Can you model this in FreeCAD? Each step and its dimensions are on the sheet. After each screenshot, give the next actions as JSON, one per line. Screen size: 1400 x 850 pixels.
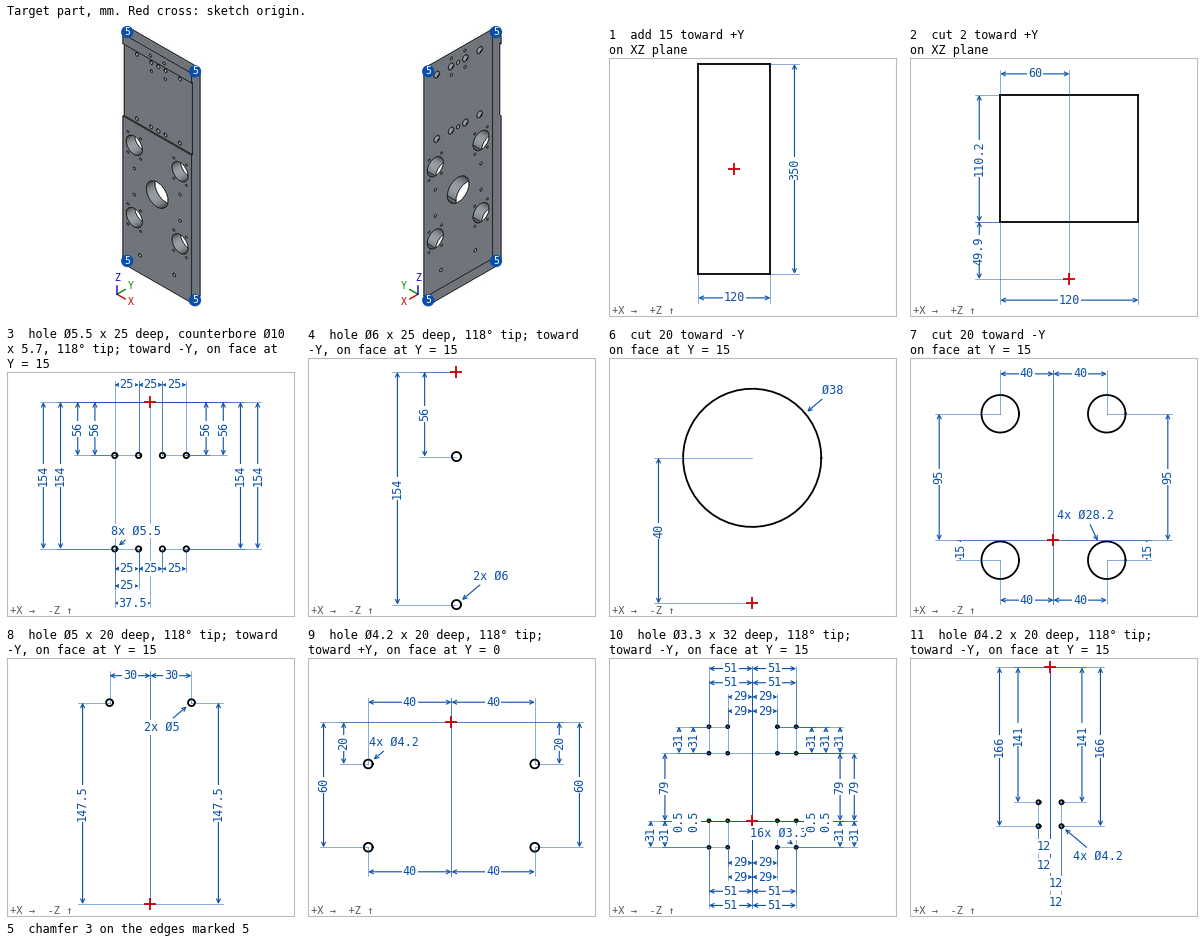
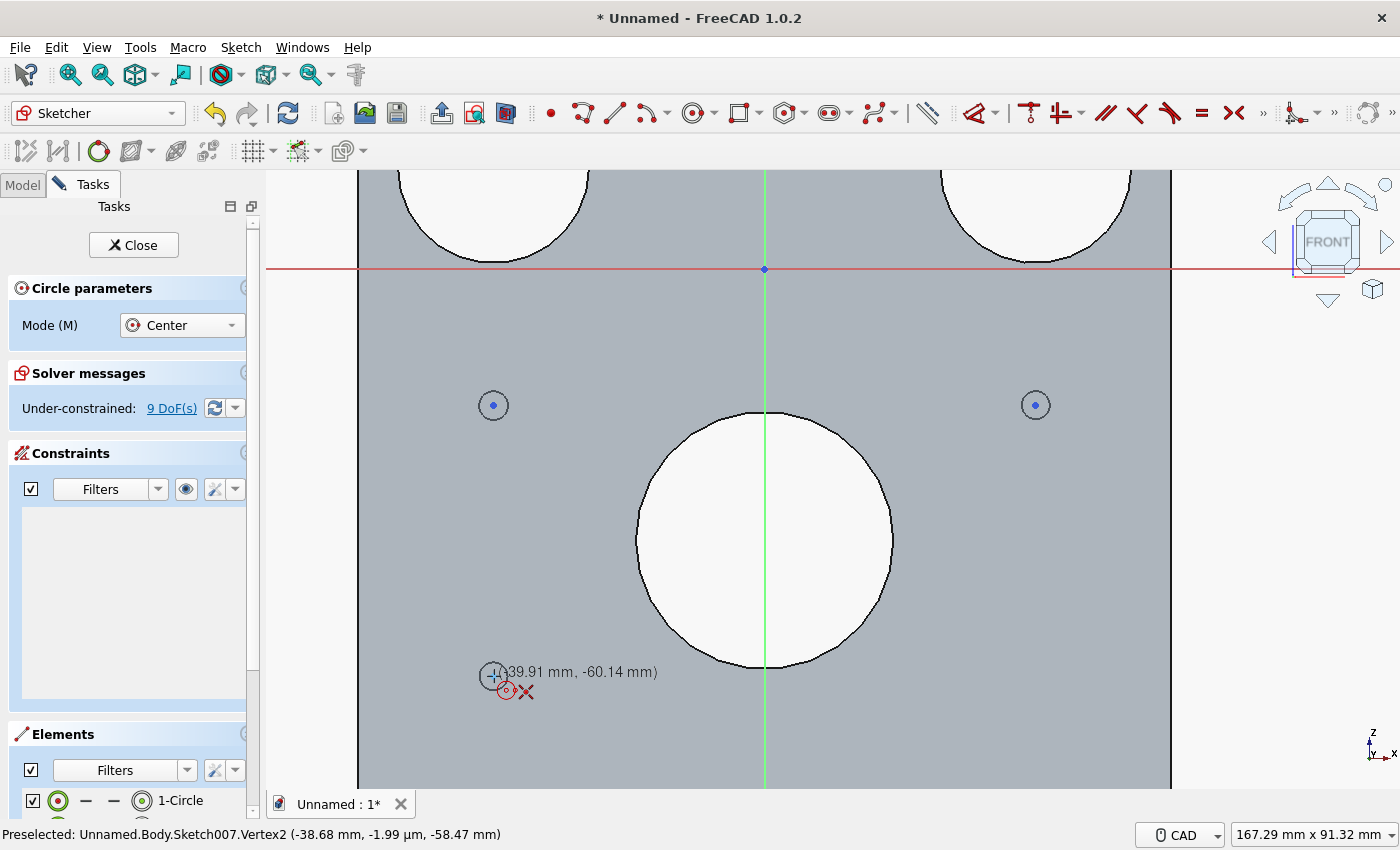
{"action": "scroll", "coordinate": [1036, 676], "scroll_direction": "up", "scroll_amount": 3}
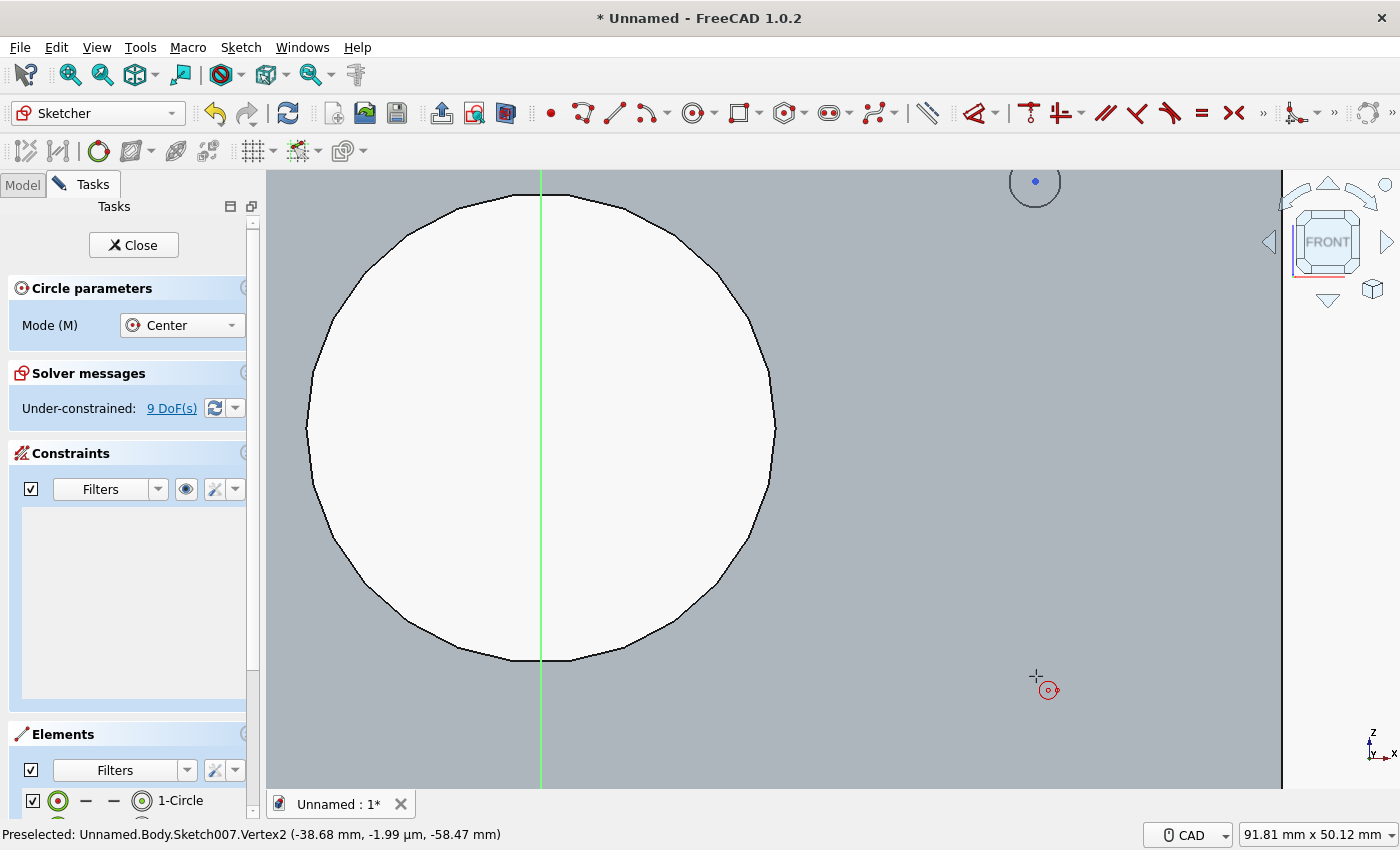
{"action": "left_click", "coordinate": [1035, 675]}
{"action": "left_click", "coordinate": [1053, 657]}
{"action": "key", "text": "Escape"}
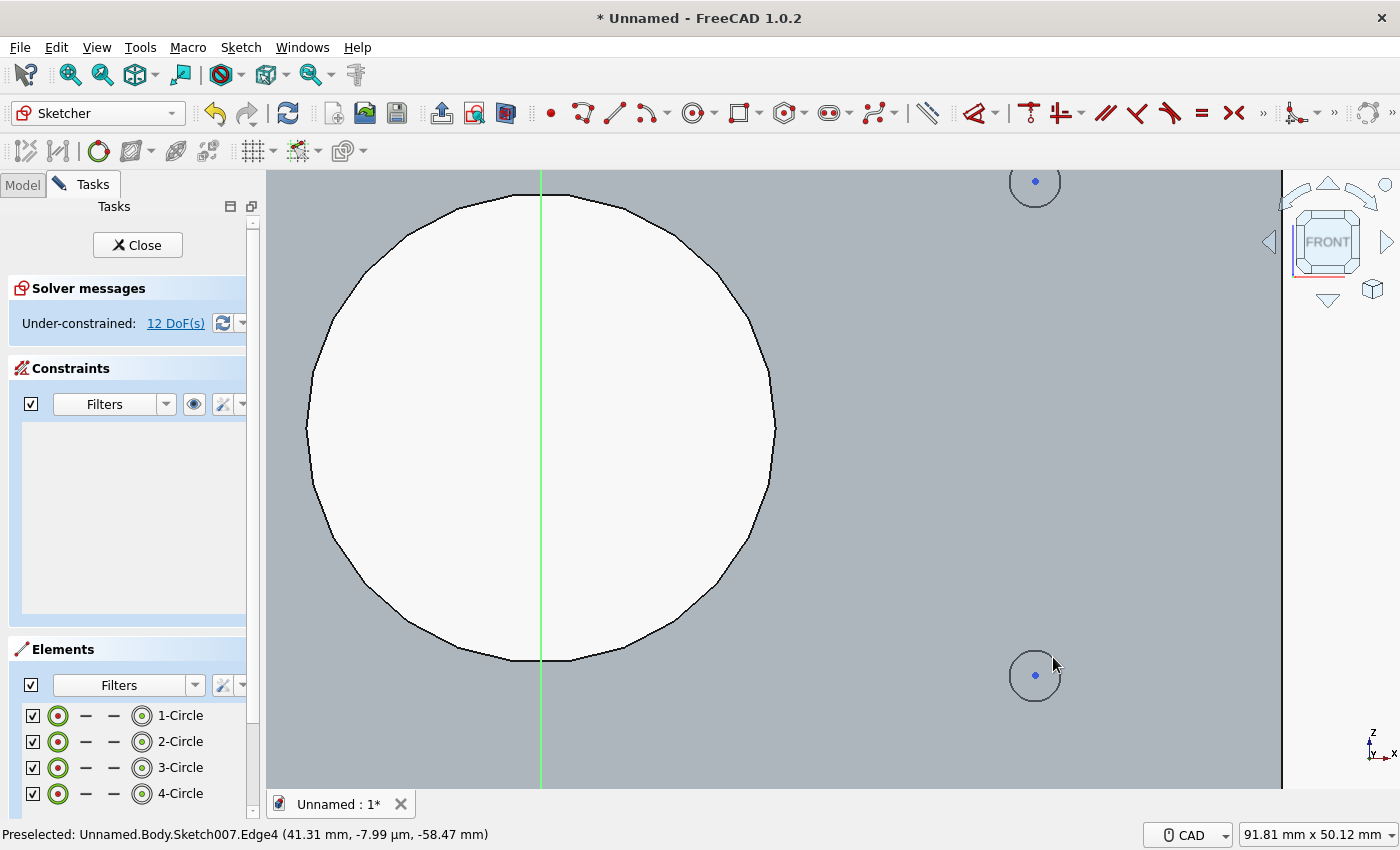
{"action": "scroll", "coordinate": [1036, 676], "scroll_direction": "down", "scroll_amount": 3}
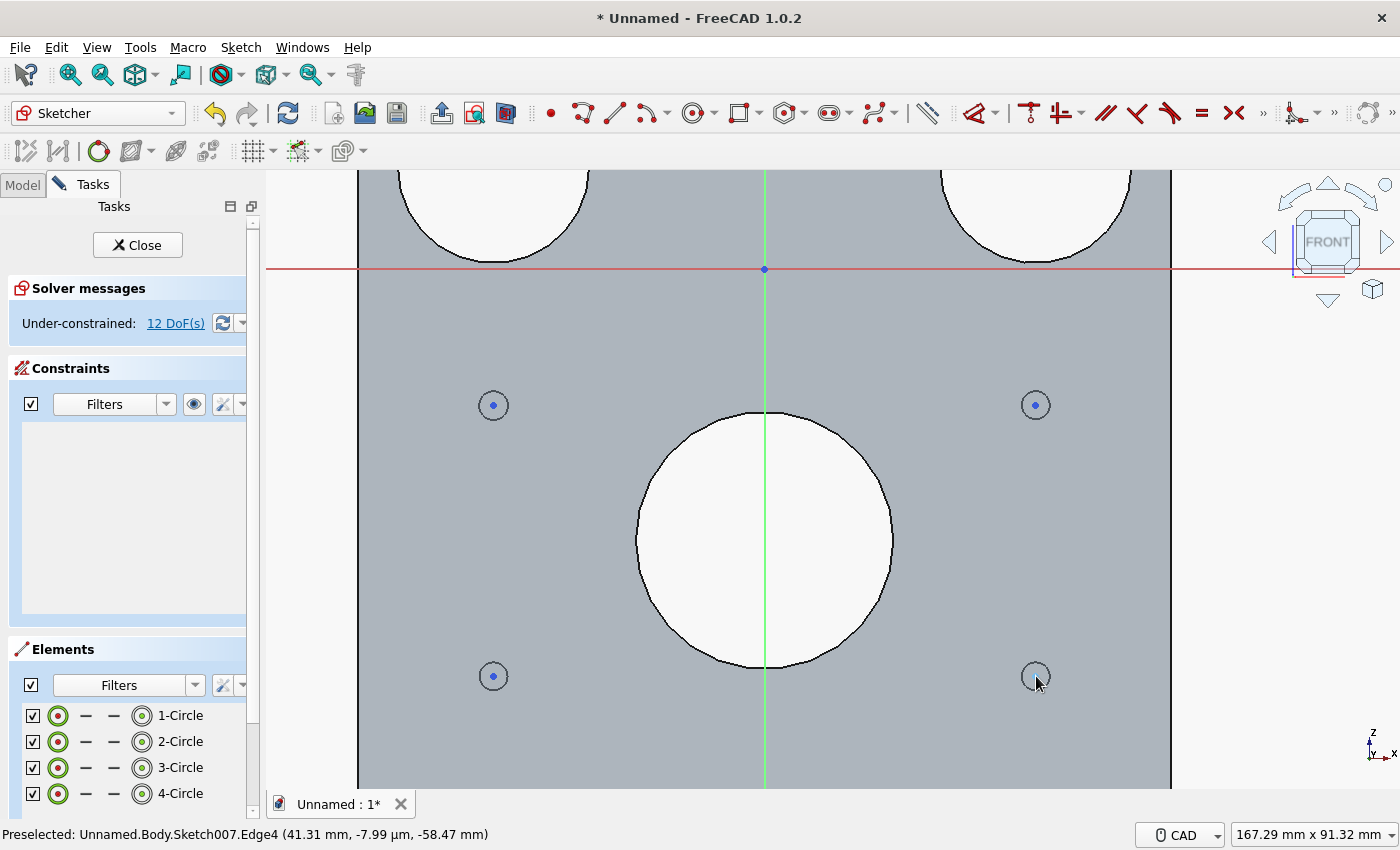
{"action": "left_click", "coordinate": [504, 395]}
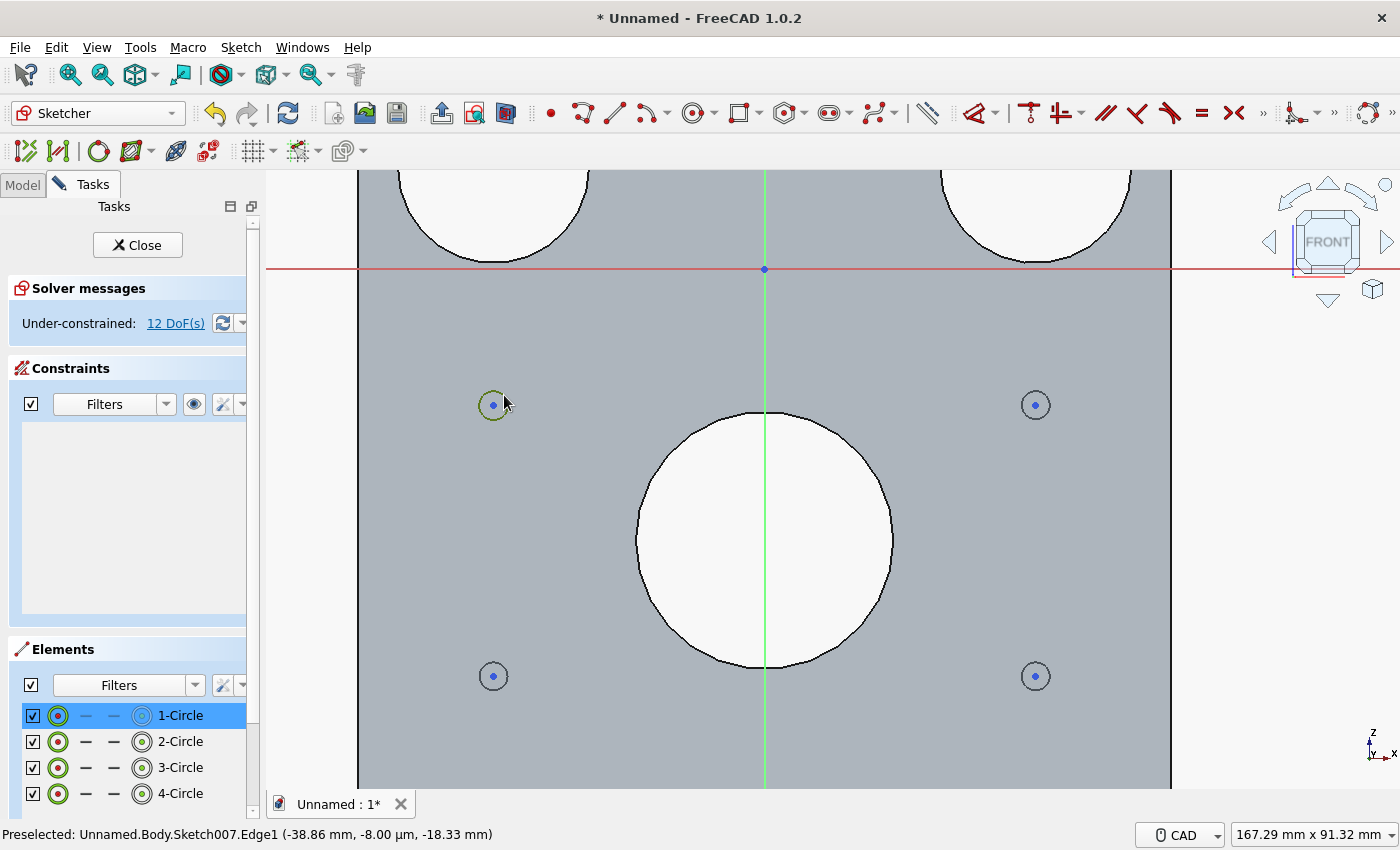
{"action": "left_click", "coordinate": [1046, 395]}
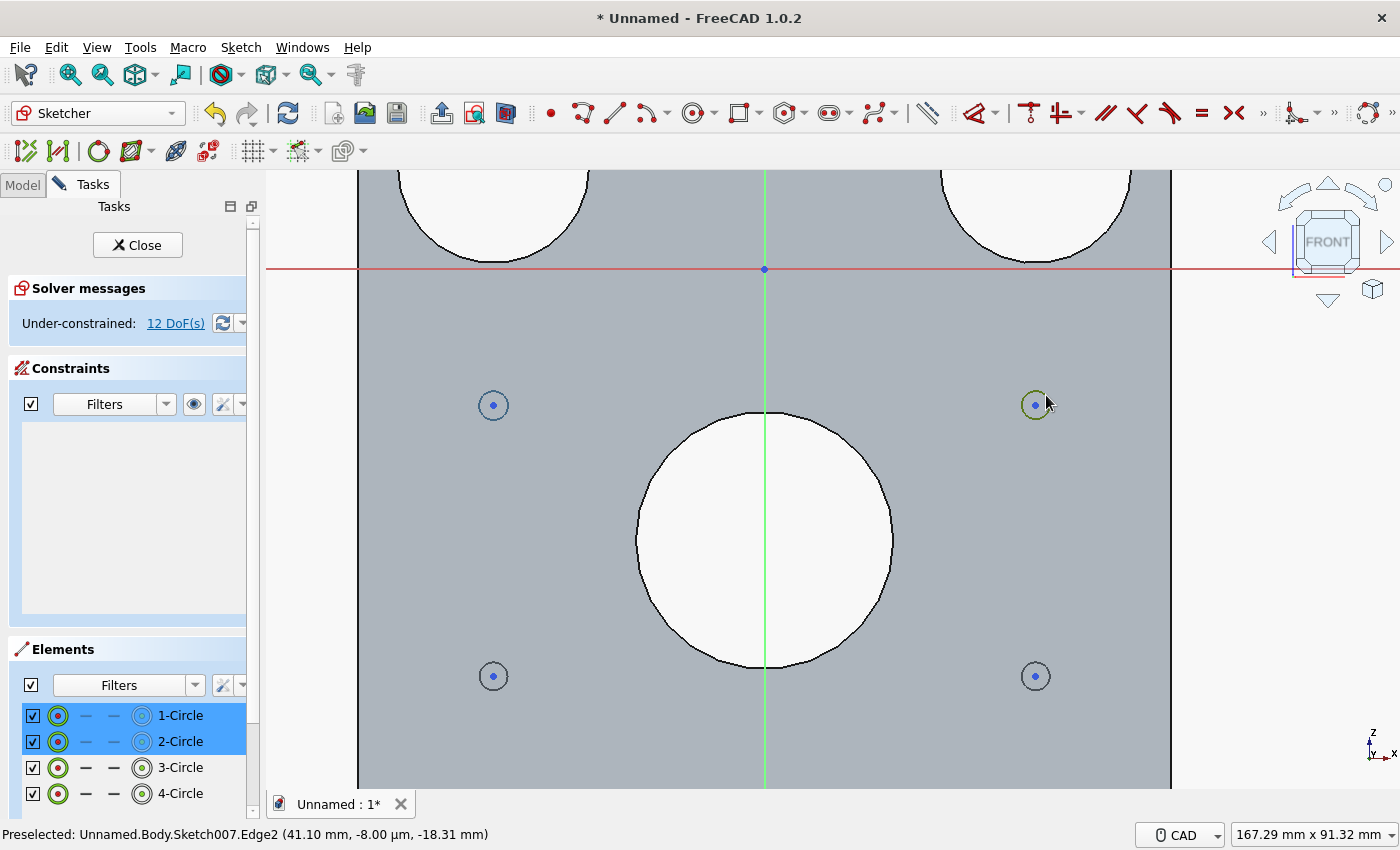
{"action": "left_click", "coordinate": [503, 666]}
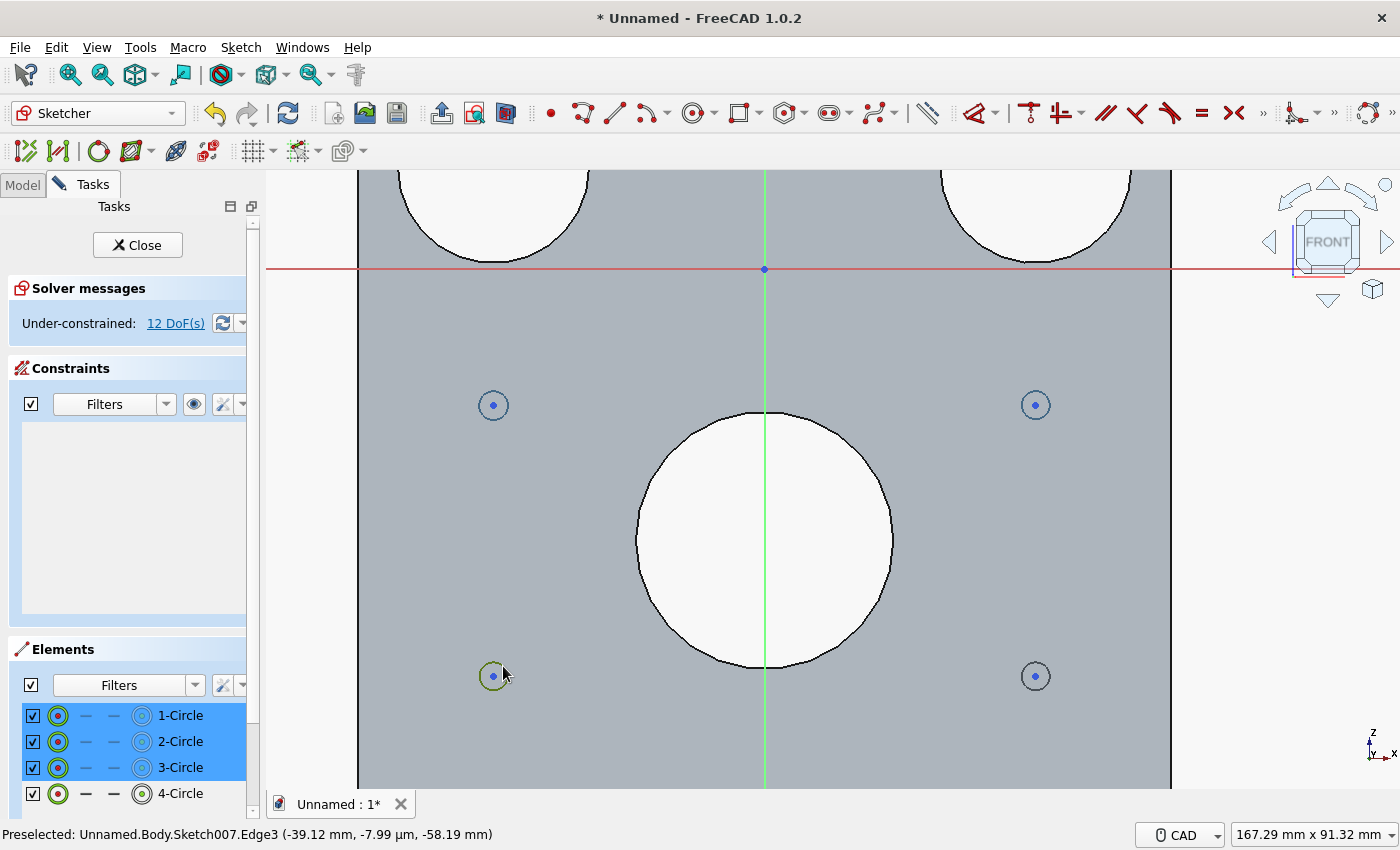
{"action": "left_click", "coordinate": [1046, 666]}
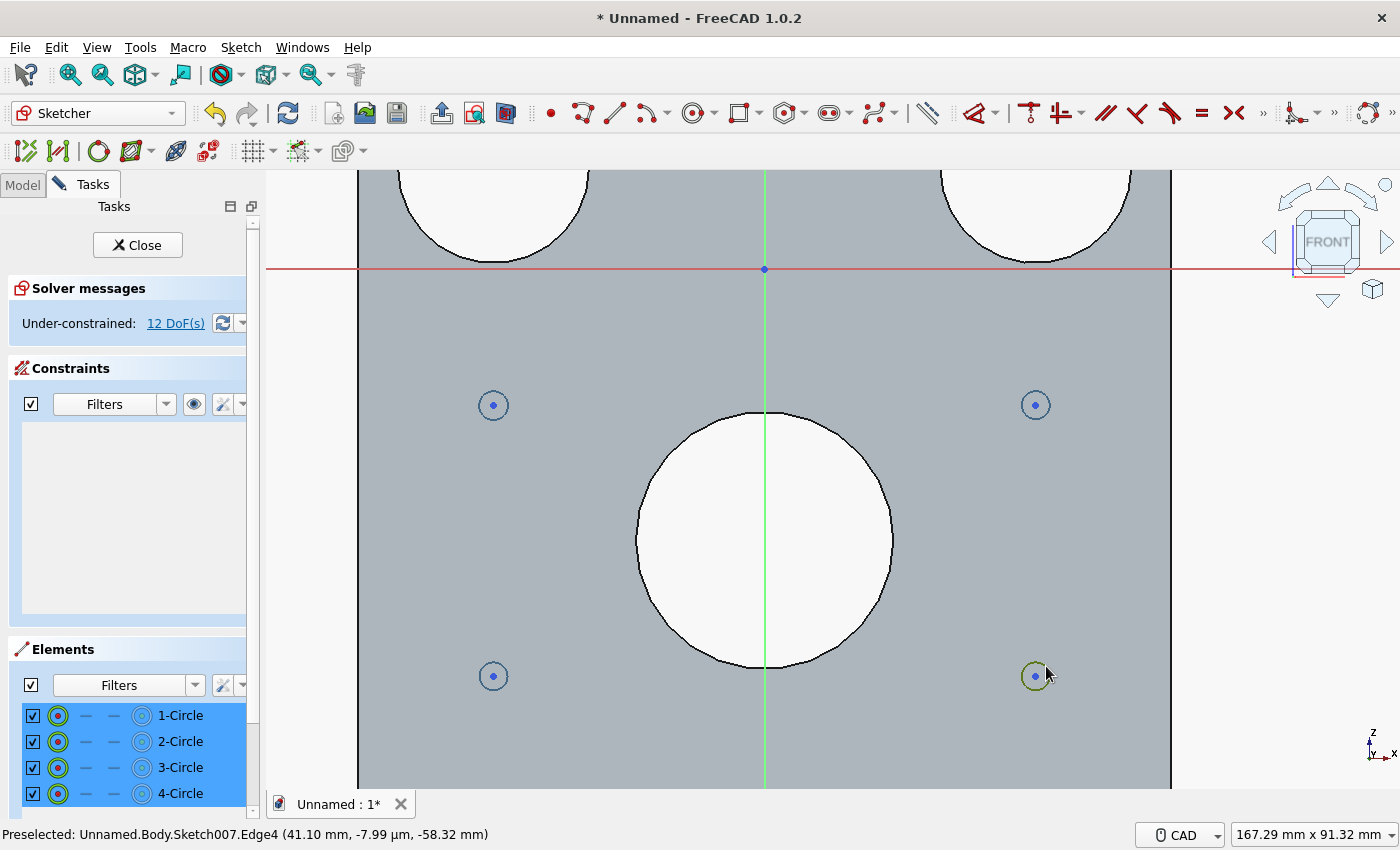
{"action": "left_click", "coordinate": [1202, 114]}